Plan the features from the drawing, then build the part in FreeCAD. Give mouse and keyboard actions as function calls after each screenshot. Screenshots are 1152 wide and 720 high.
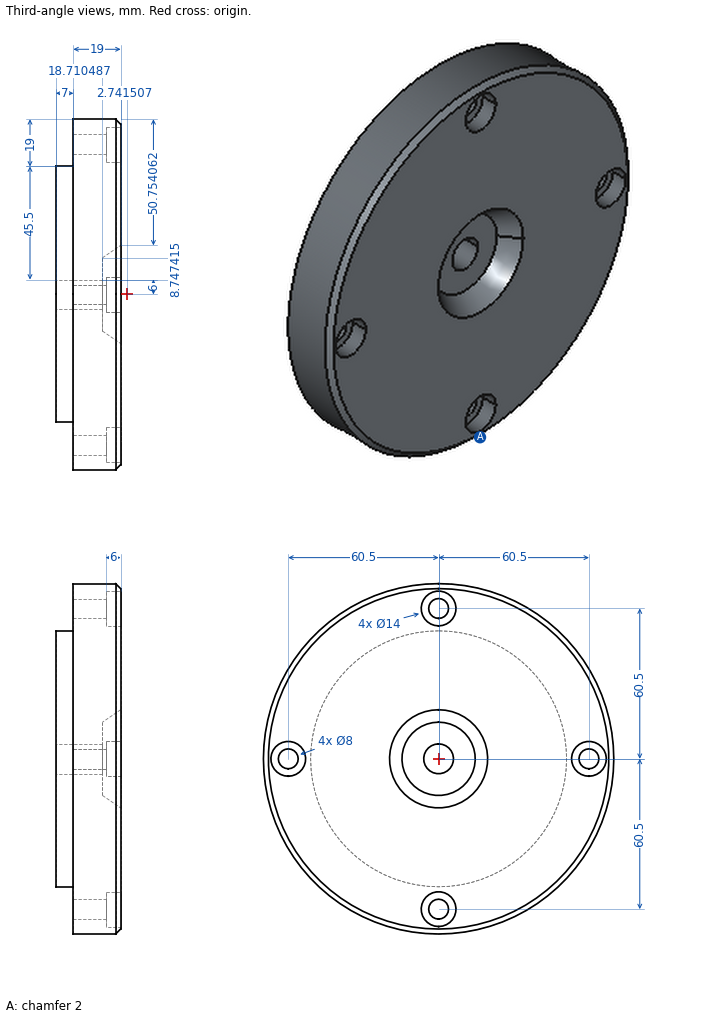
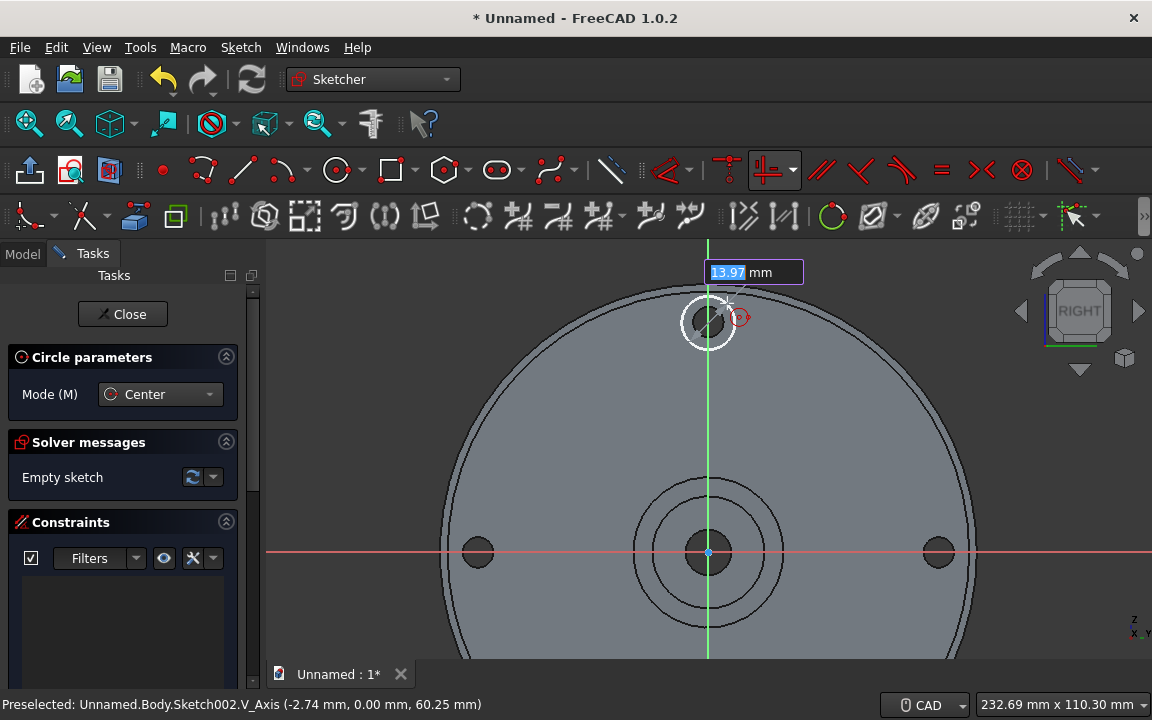
text(14)
key(Return)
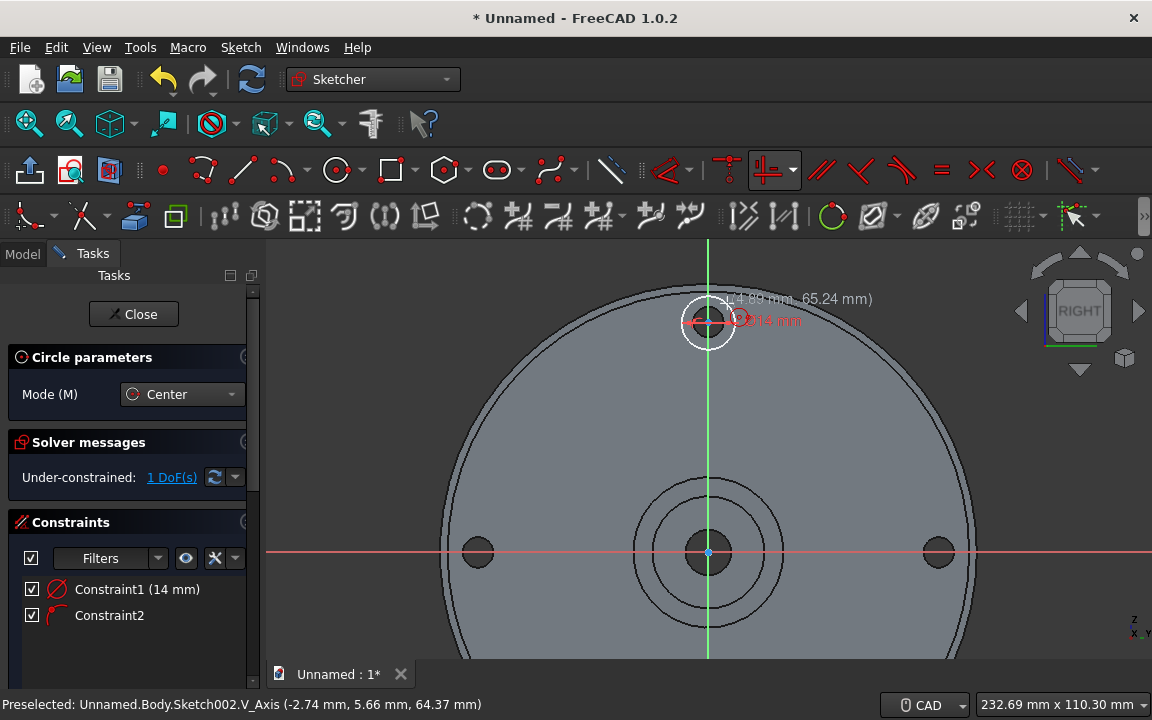
click(939, 552)
move(958, 534)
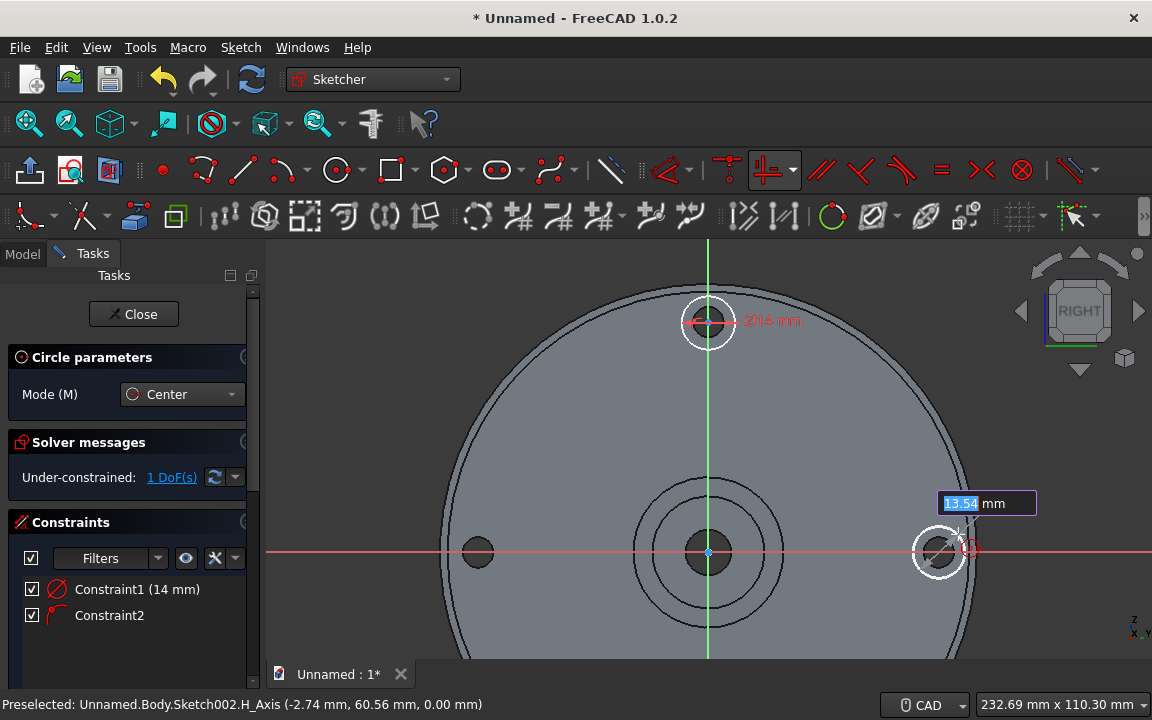
text(14)
key(Return)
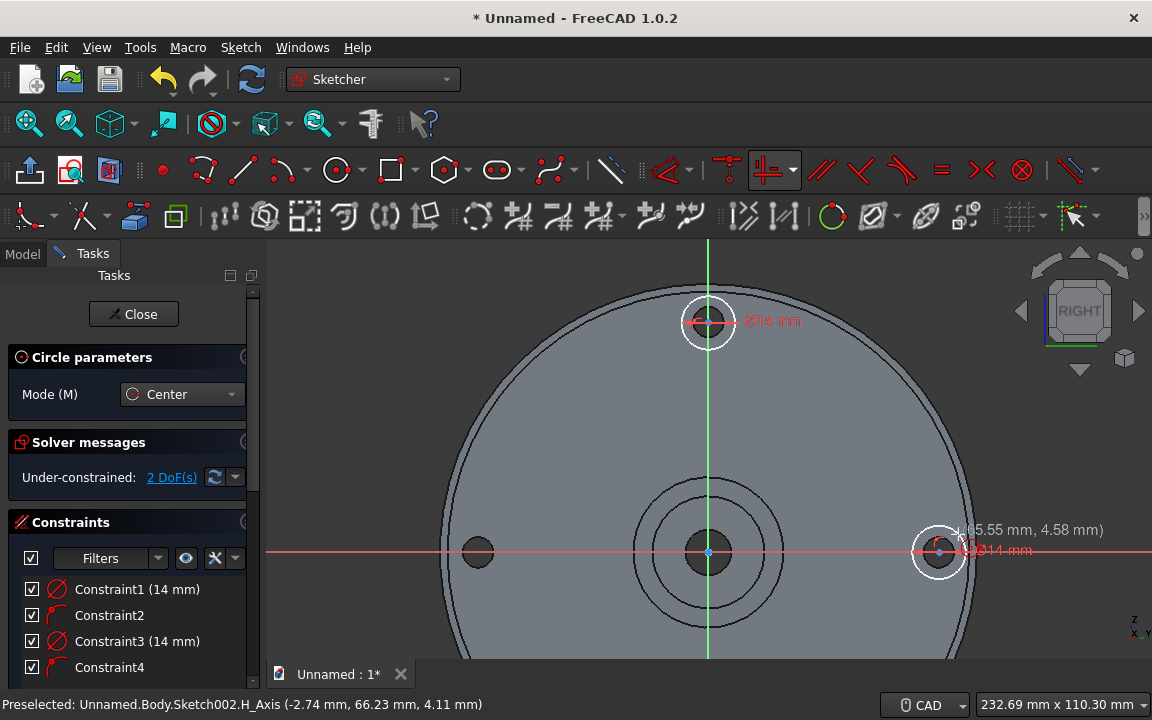
scroll(558, 323, down, 3)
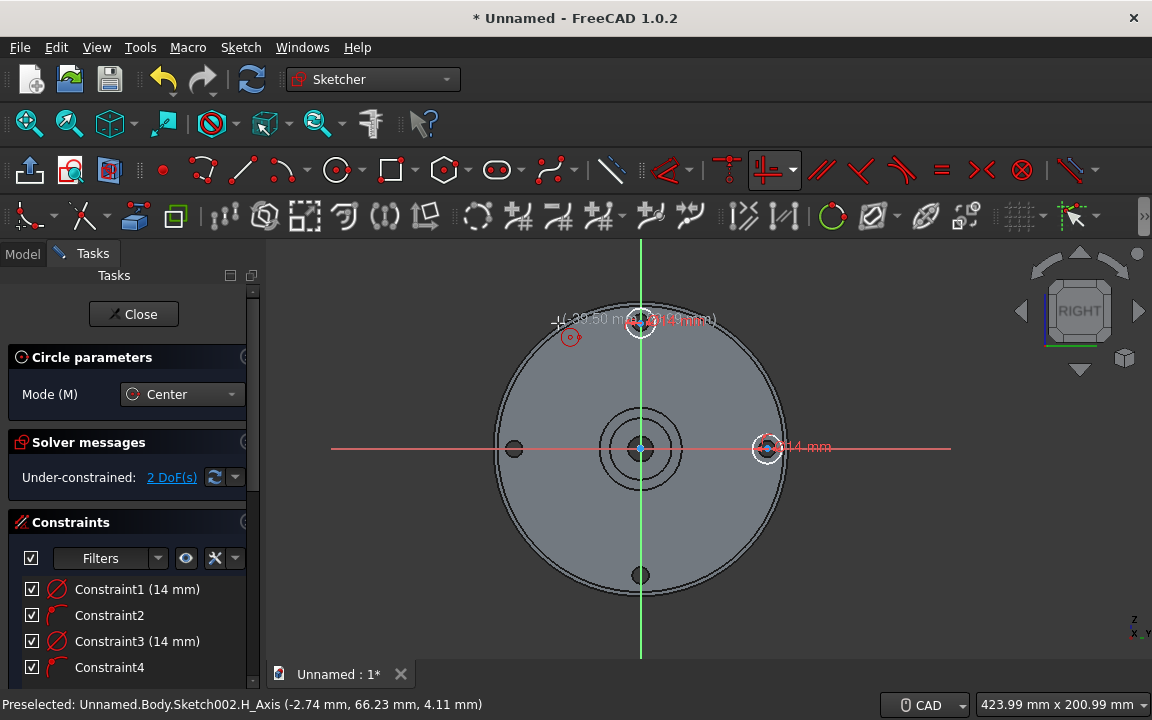
scroll(641, 575, up, 3)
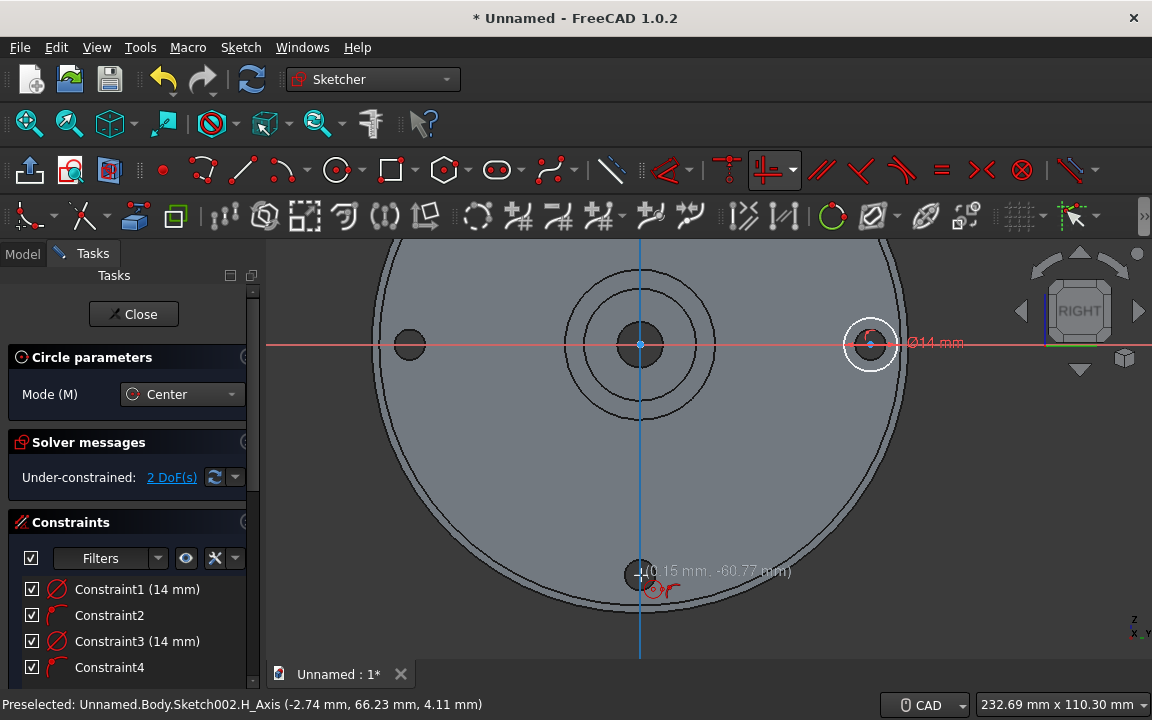
click(640, 575)
move(659, 556)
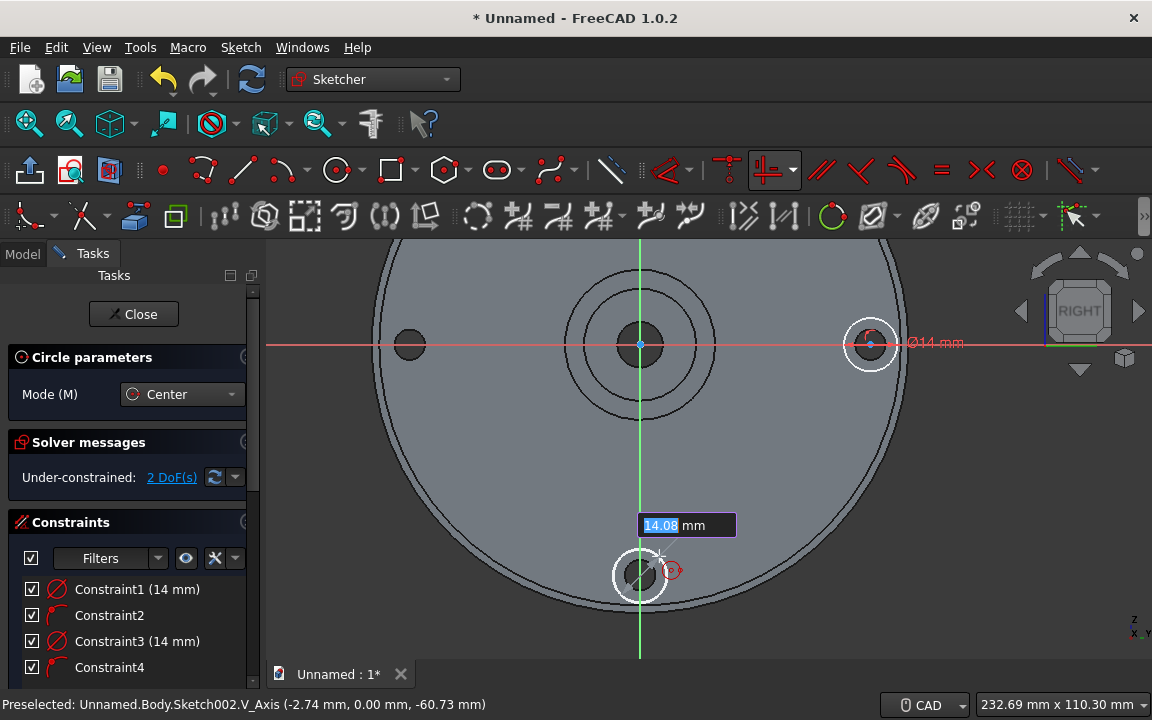
text(14)
key(Return)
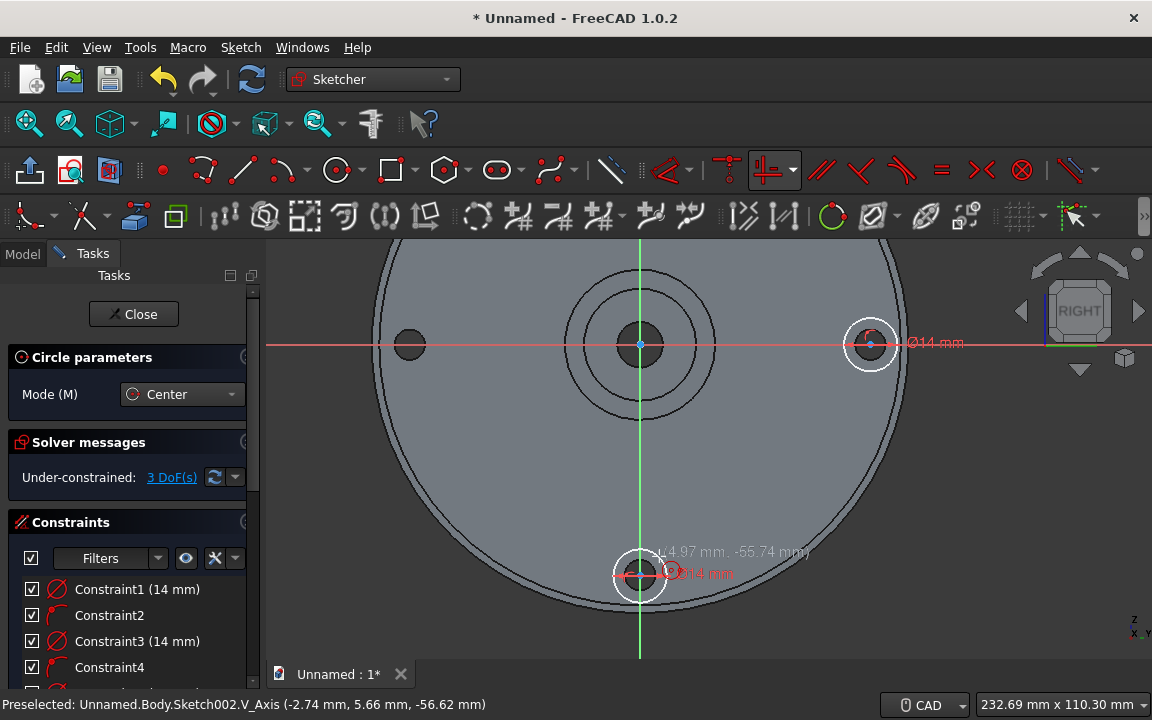
click(410, 345)
move(429, 326)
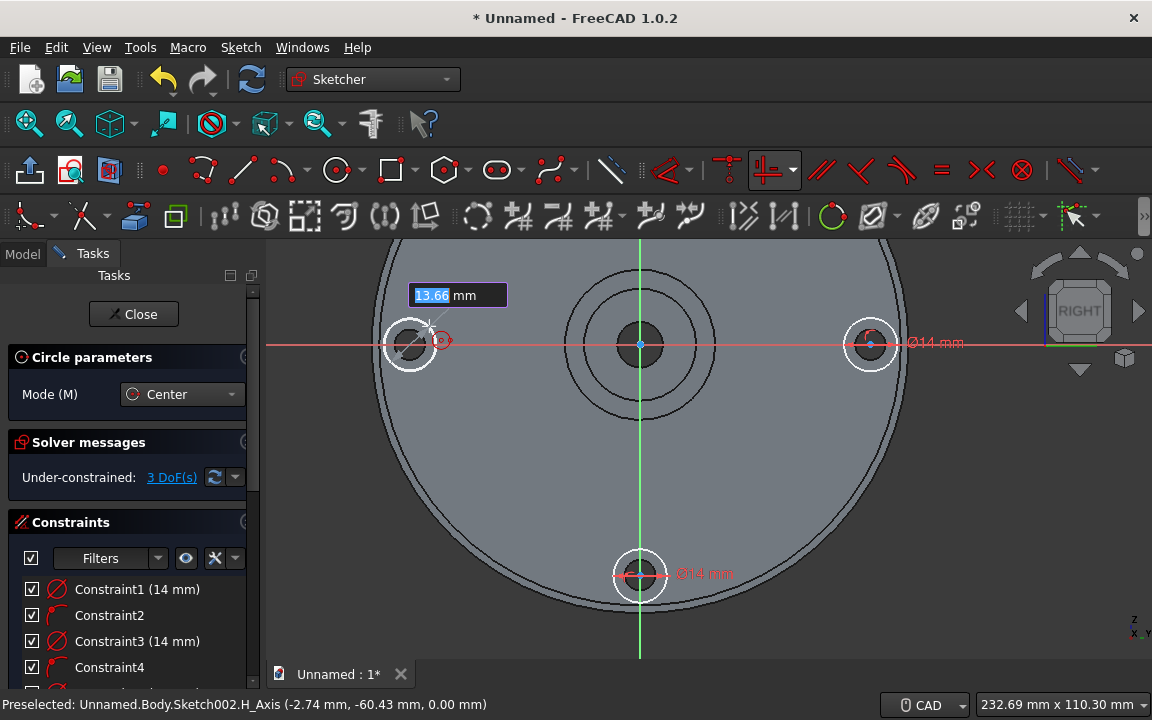
text(14)
key(Return)
key(Escape)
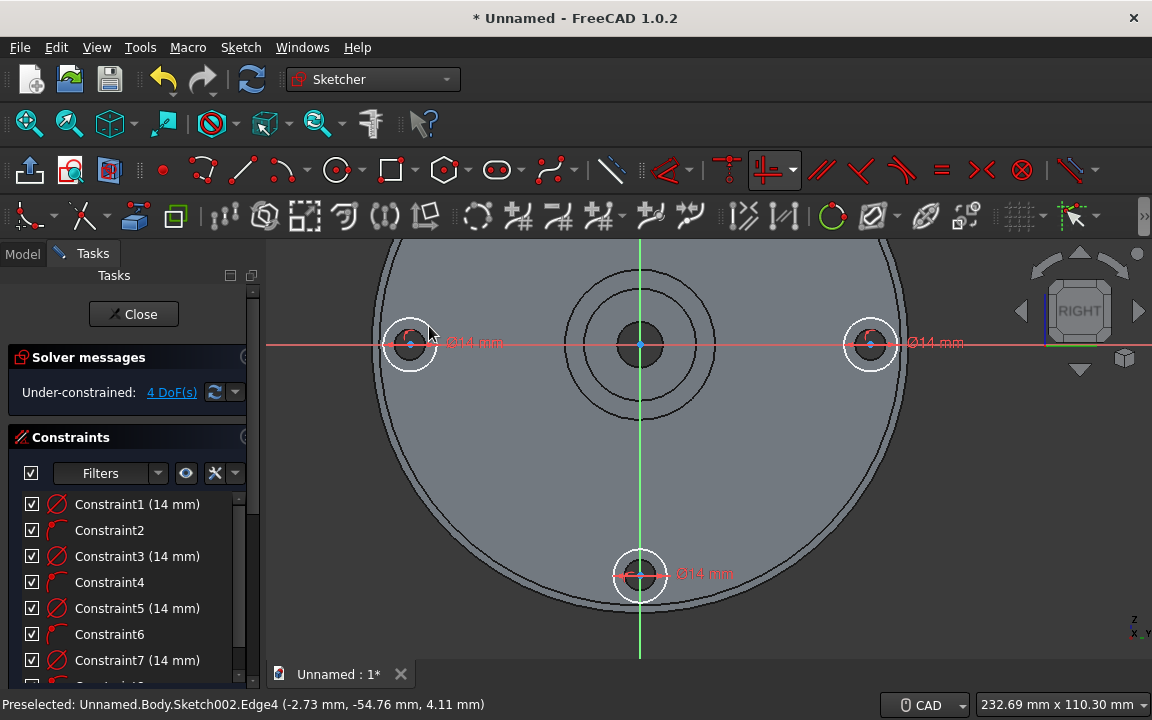
click(666, 170)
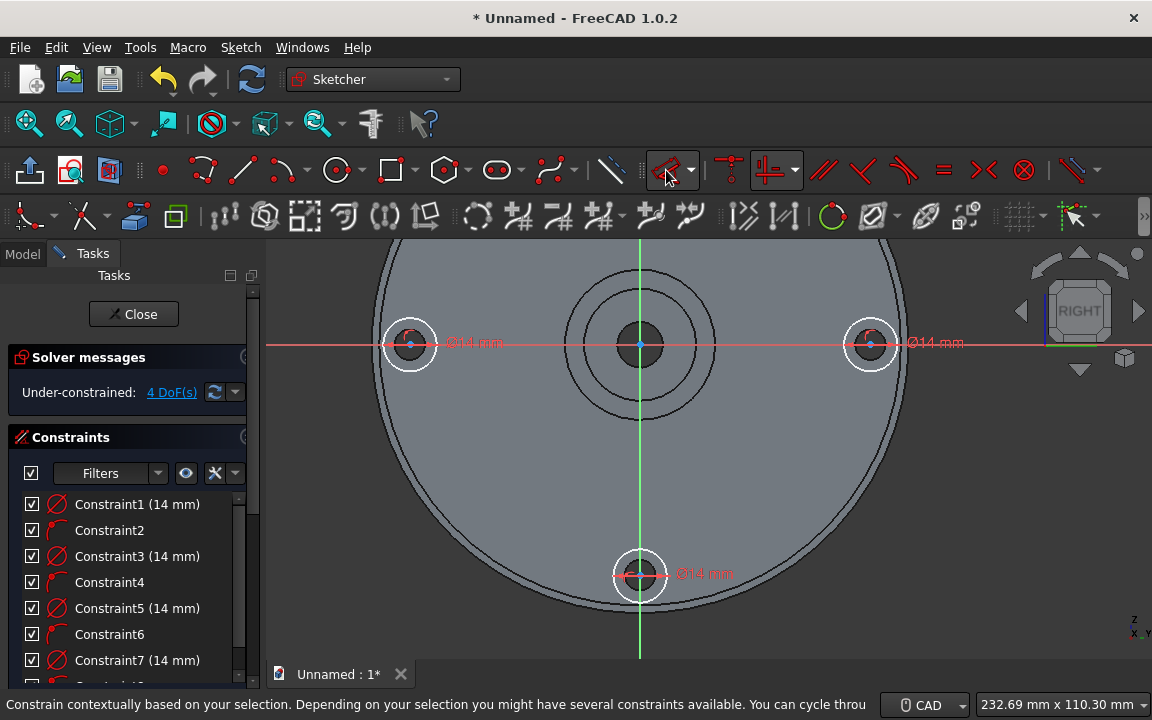
scroll(641, 576, down, 3)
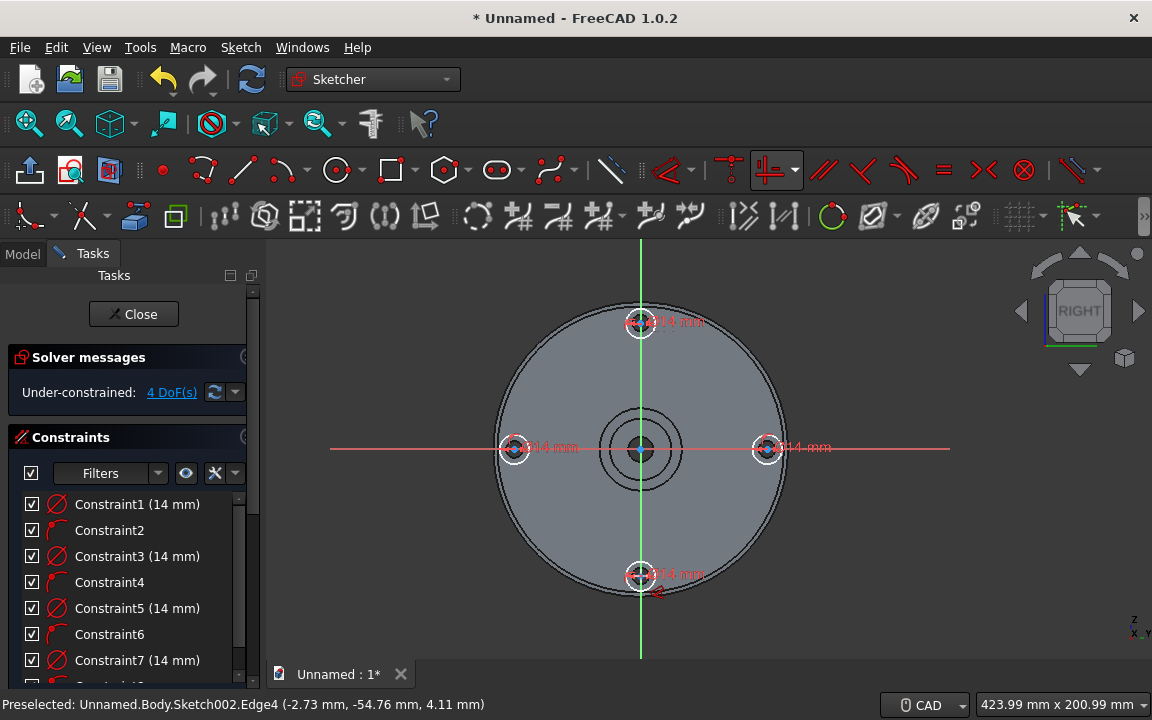
click(641, 324)
click(675, 386)